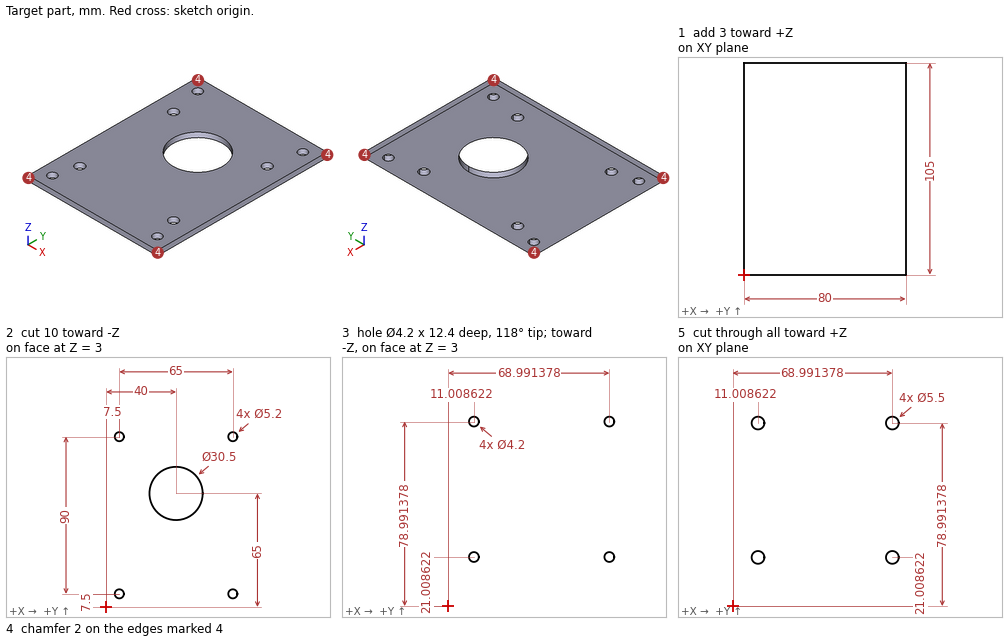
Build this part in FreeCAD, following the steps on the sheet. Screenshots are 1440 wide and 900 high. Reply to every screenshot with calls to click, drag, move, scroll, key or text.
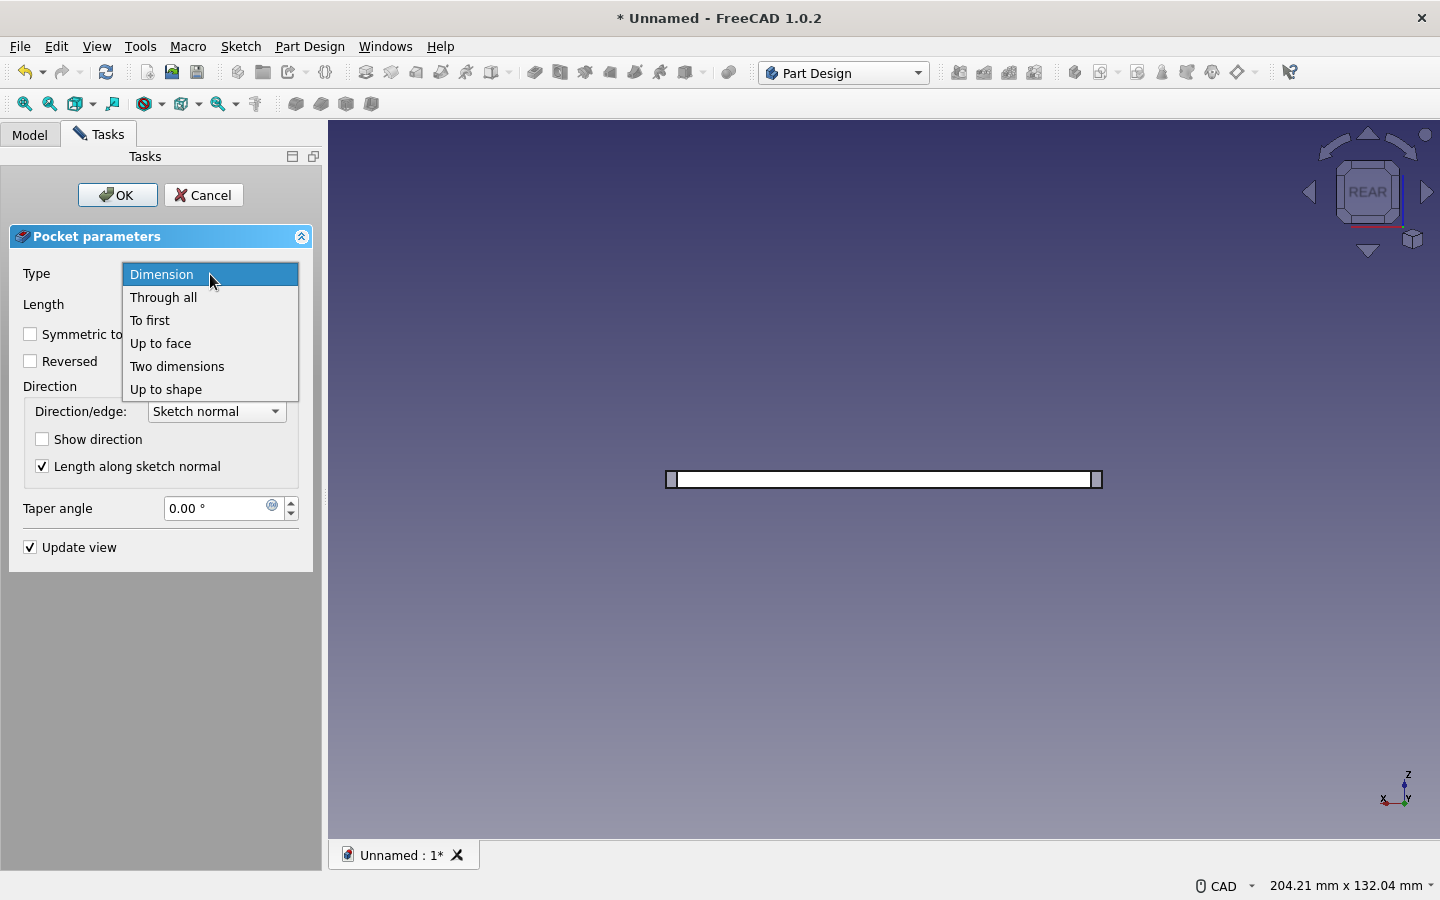
click(208, 298)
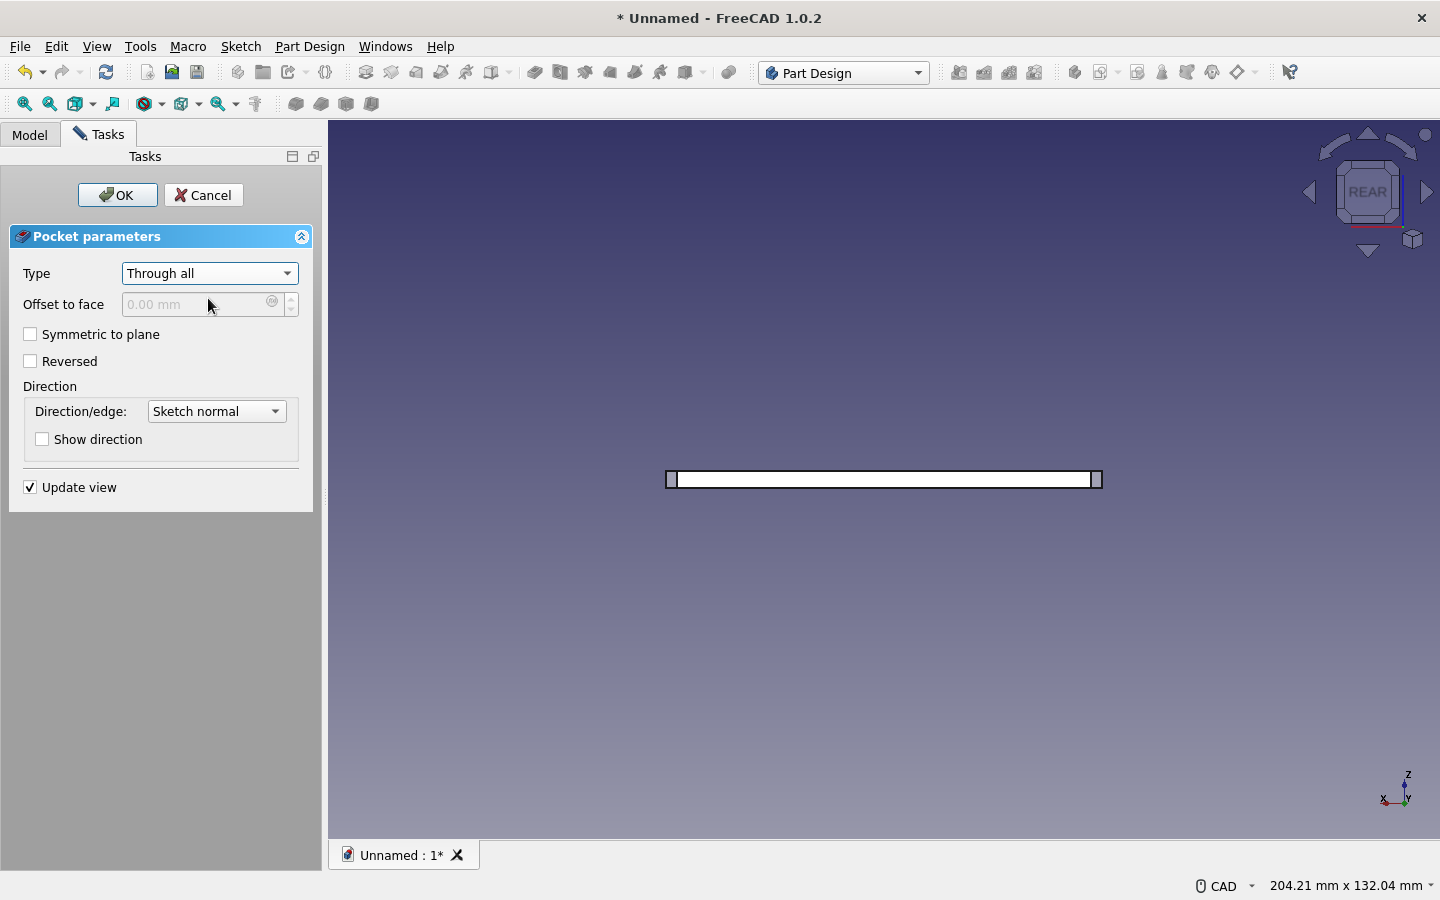
click(31, 361)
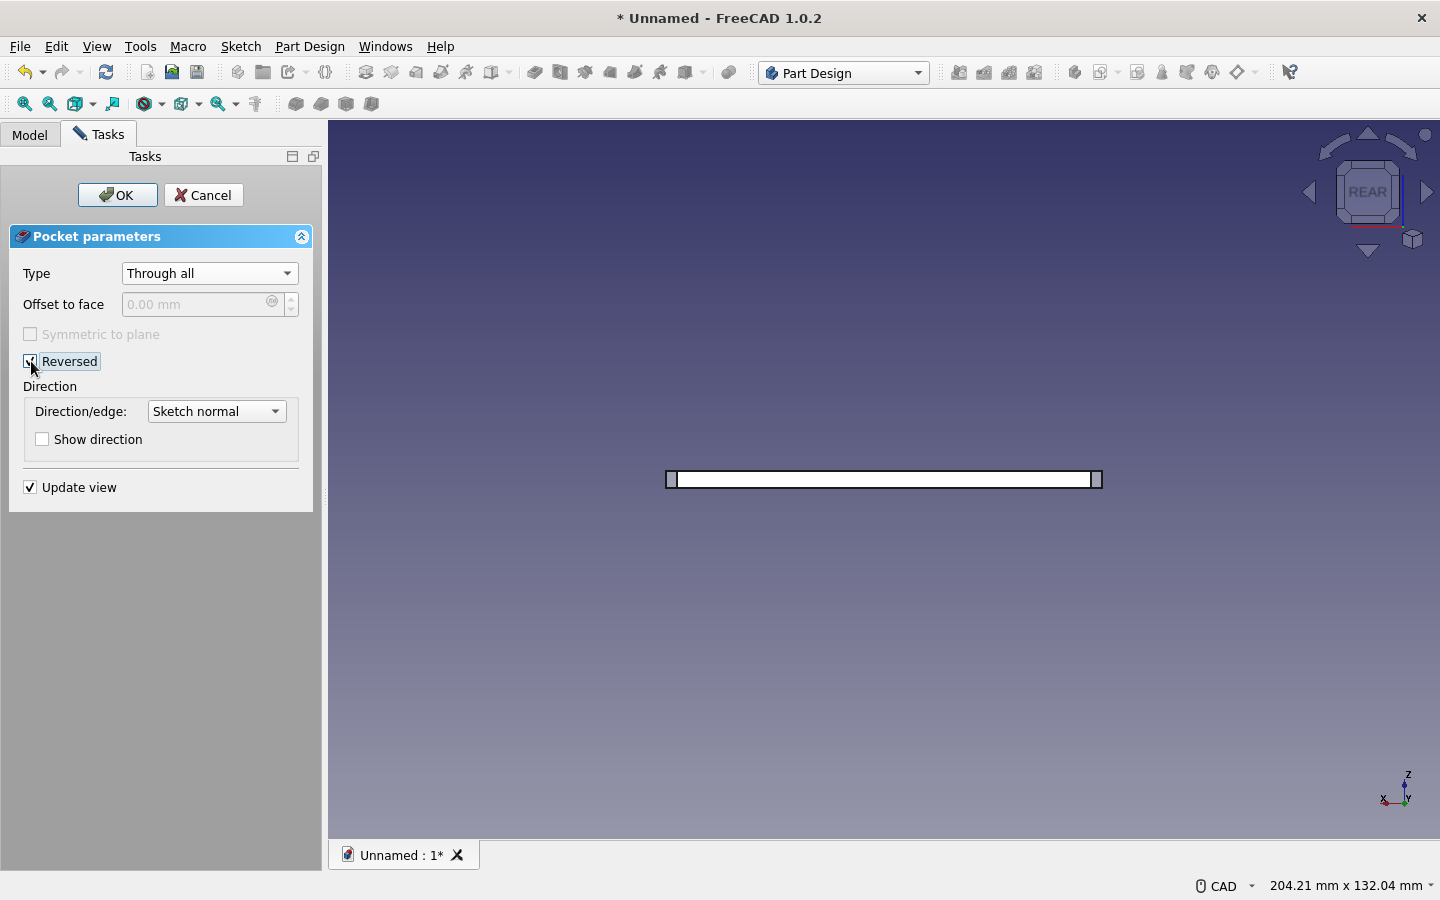
click(118, 195)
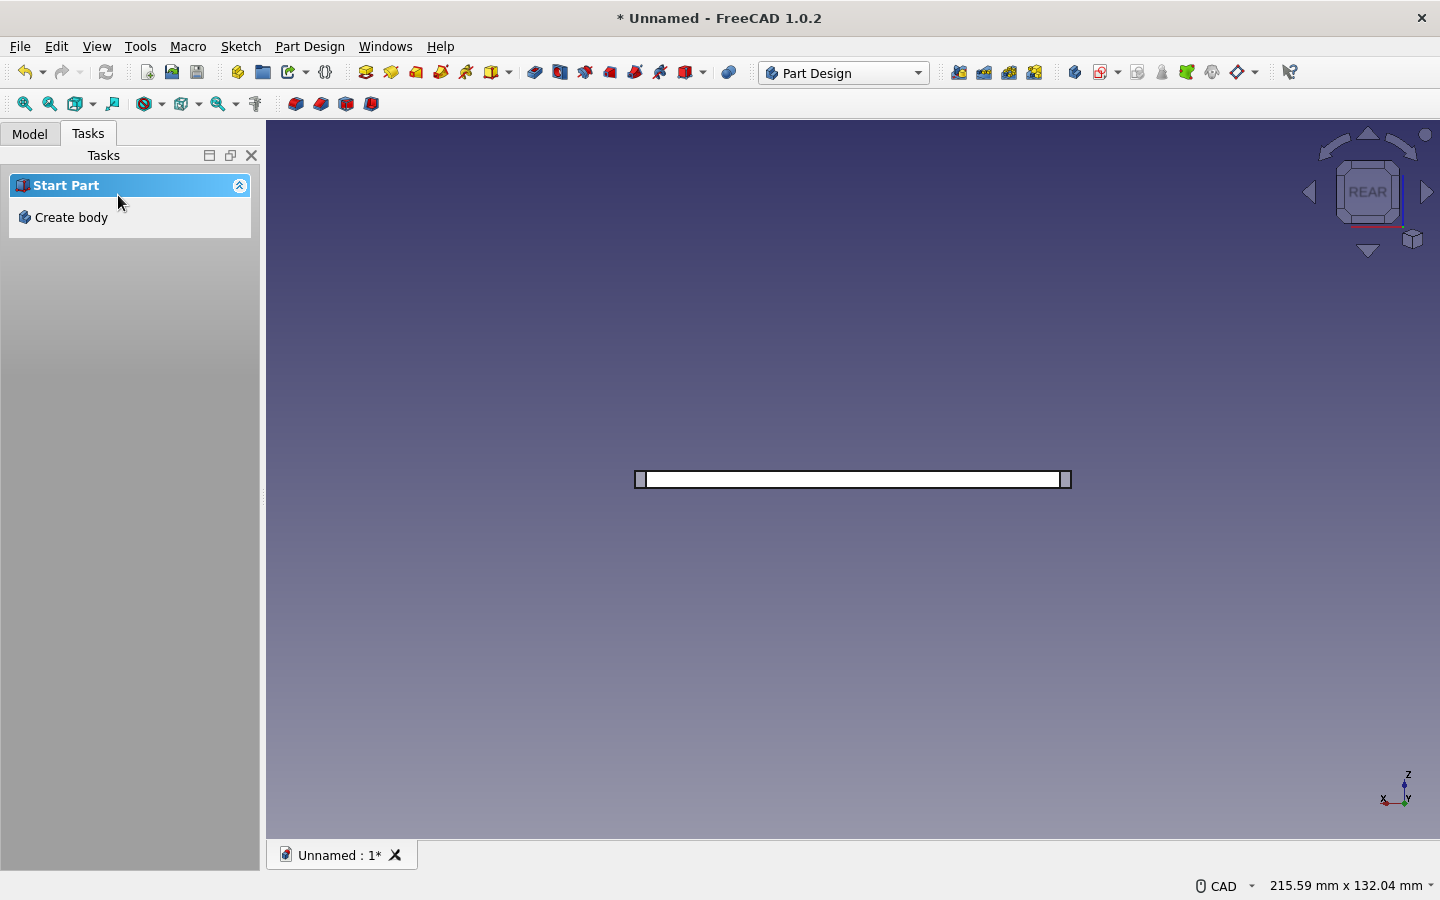
key(0)